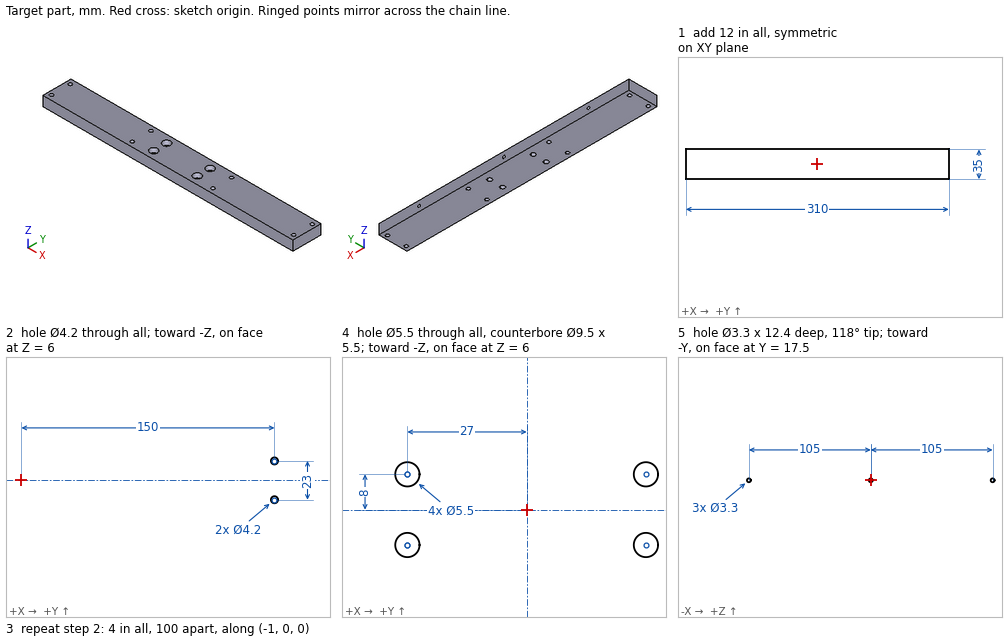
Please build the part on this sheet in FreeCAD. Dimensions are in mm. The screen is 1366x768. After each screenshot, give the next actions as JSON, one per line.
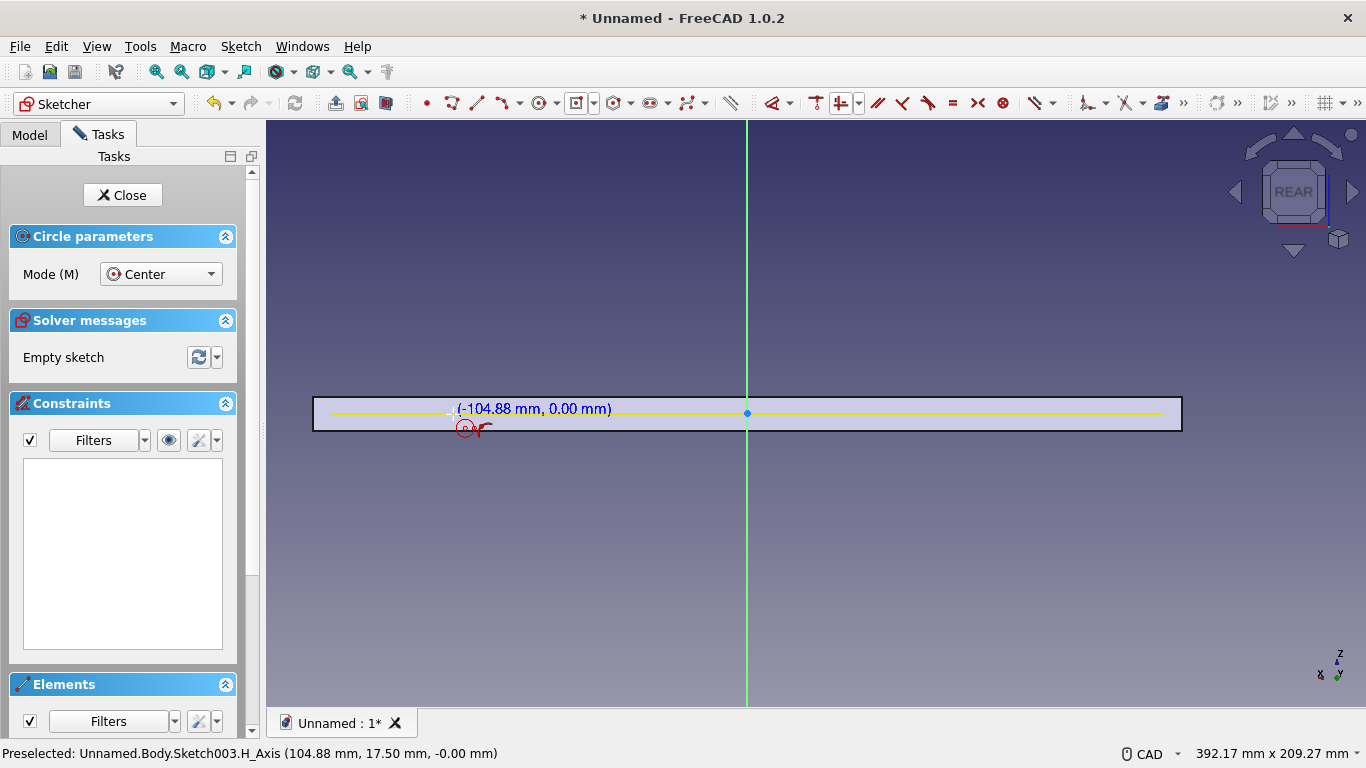
{"action": "left_click", "coordinate": [453, 414]}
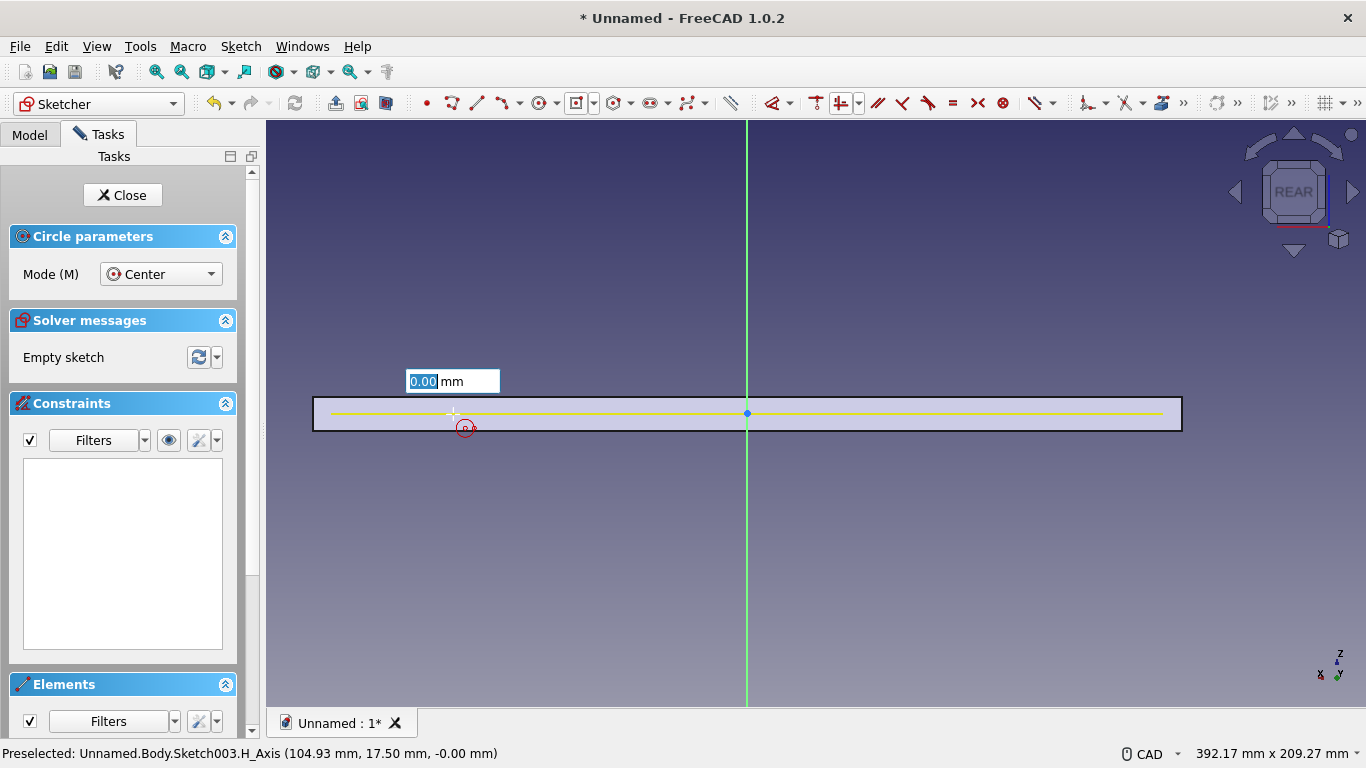
{"action": "scroll", "coordinate": [451, 418], "scroll_direction": "up", "scroll_amount": 7}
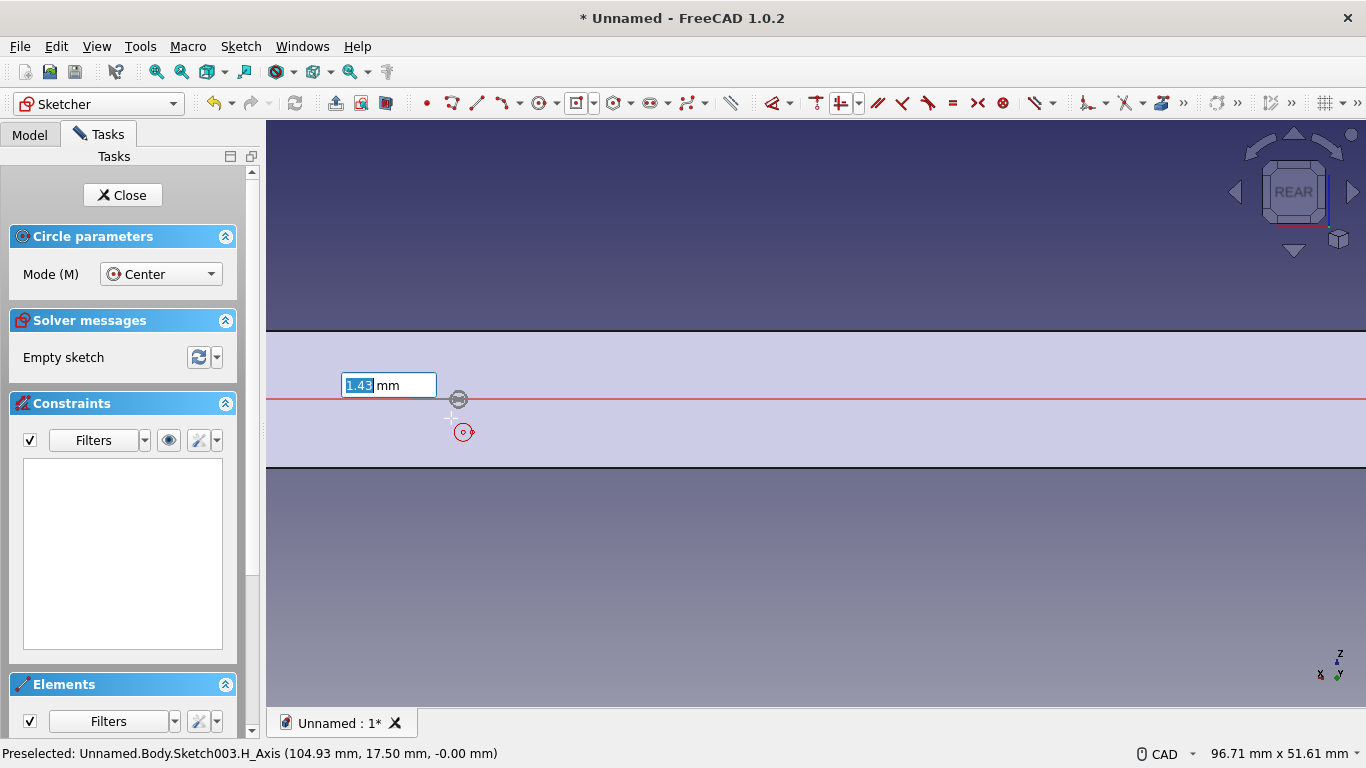
{"action": "left_click", "coordinate": [451, 417]}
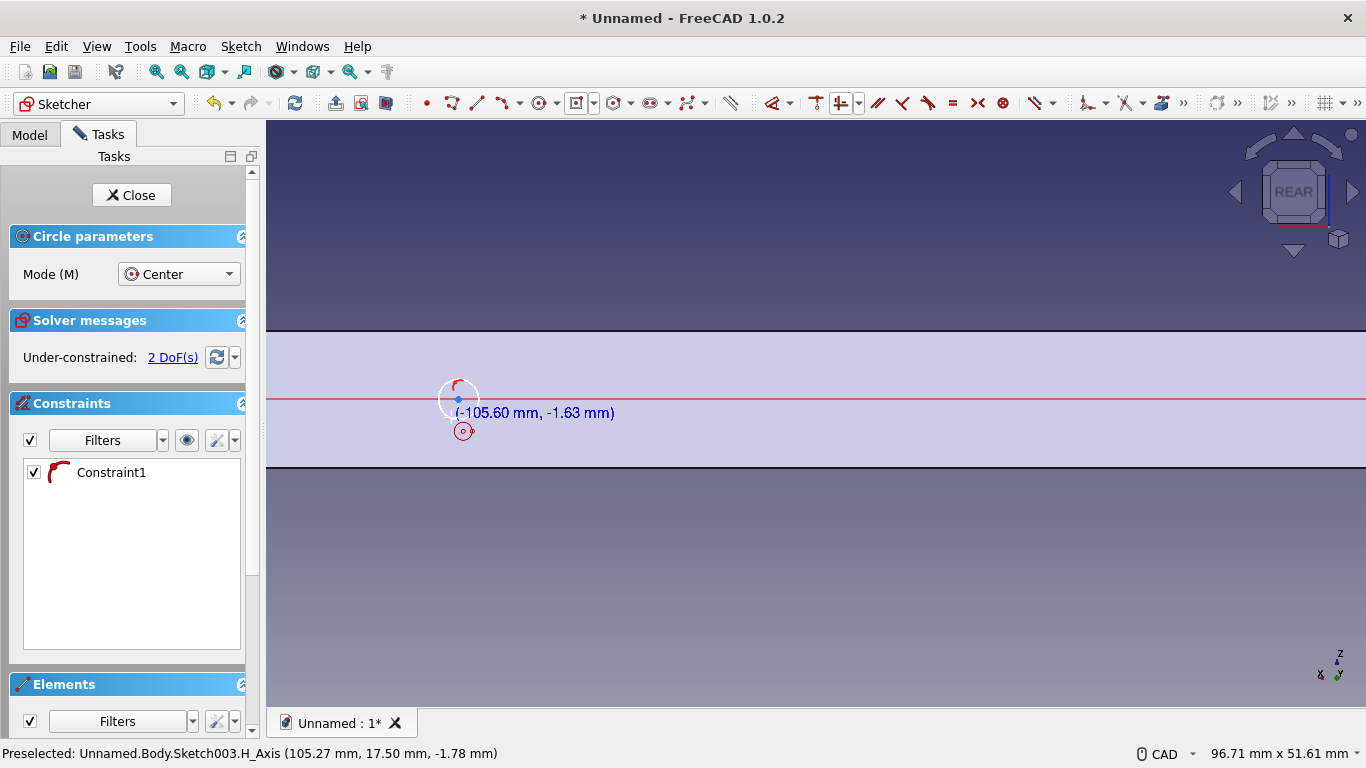
{"action": "scroll", "coordinate": [451, 418], "scroll_direction": "down", "scroll_amount": 7}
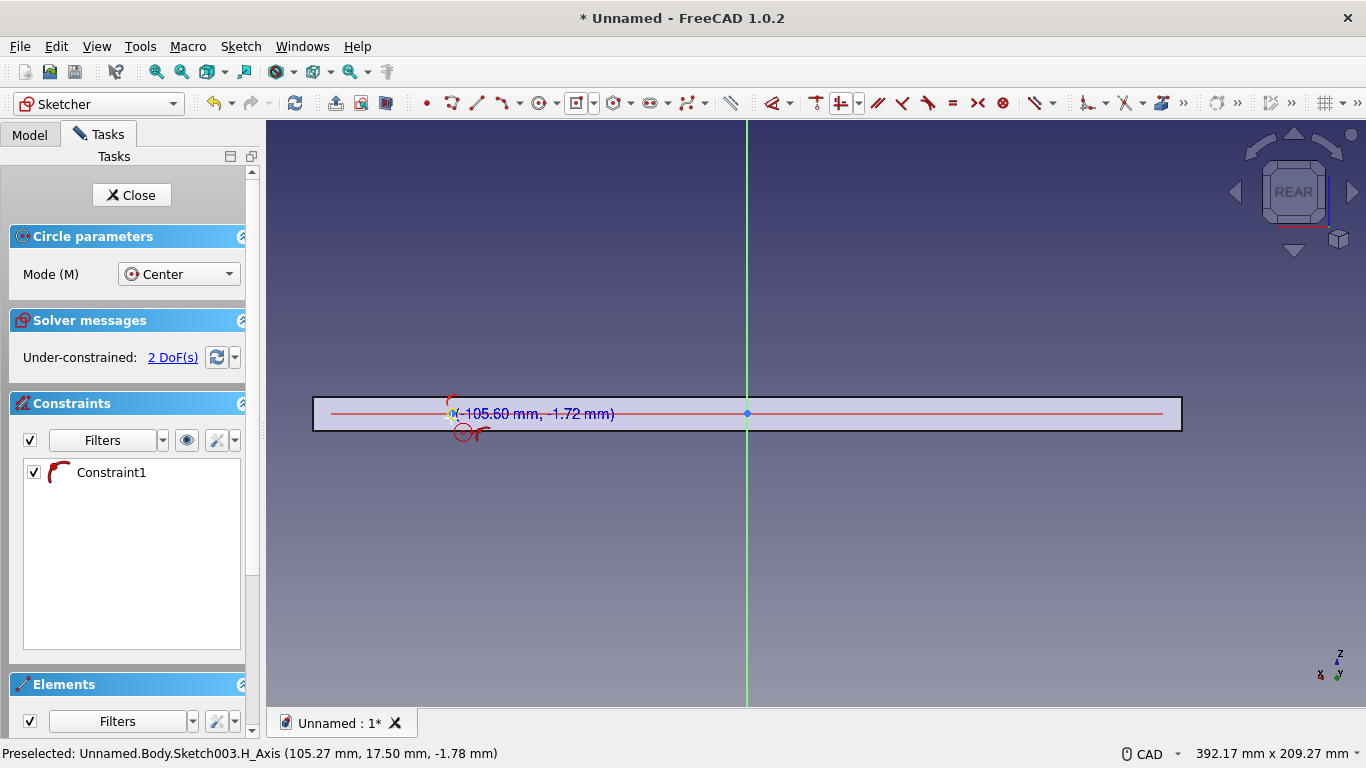
{"action": "scroll", "coordinate": [747, 414], "scroll_direction": "up", "scroll_amount": 8}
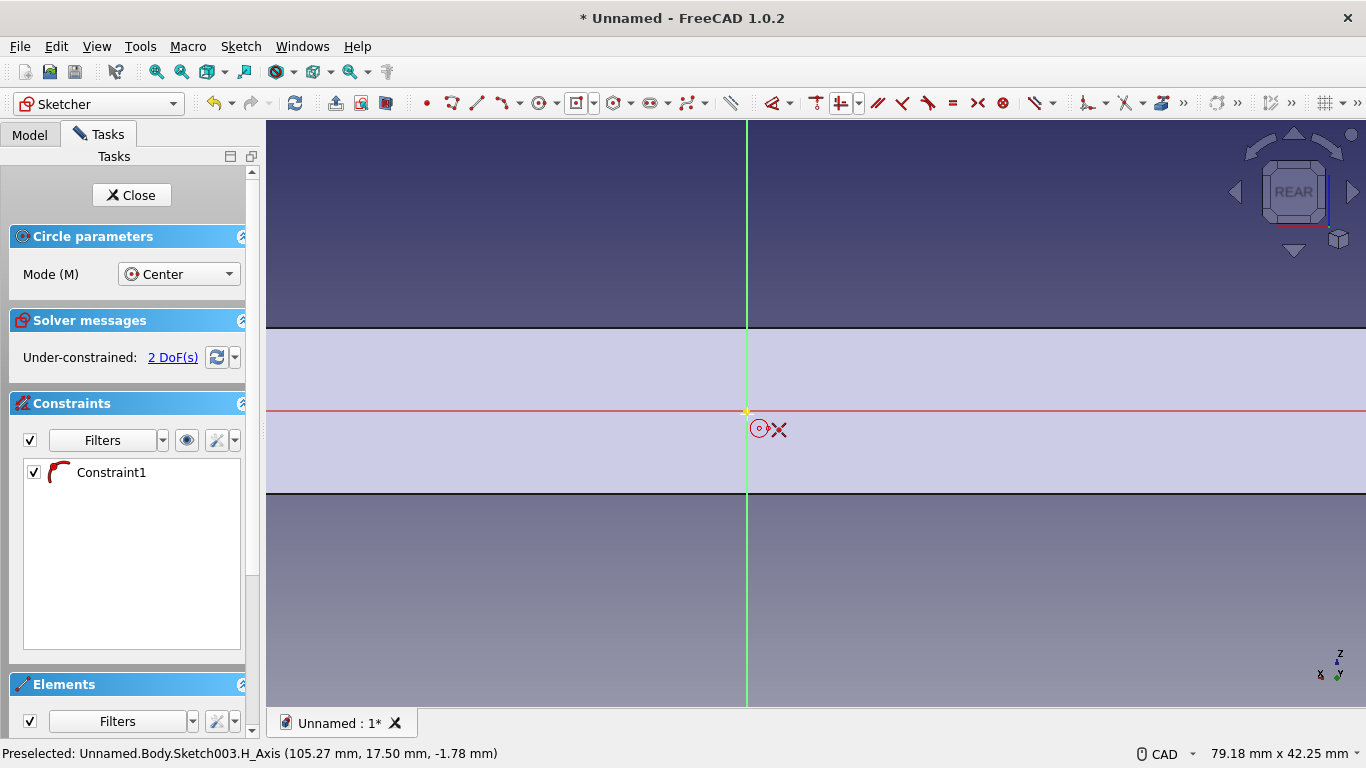
{"action": "scroll", "coordinate": [748, 414], "scroll_direction": "down", "scroll_amount": 8}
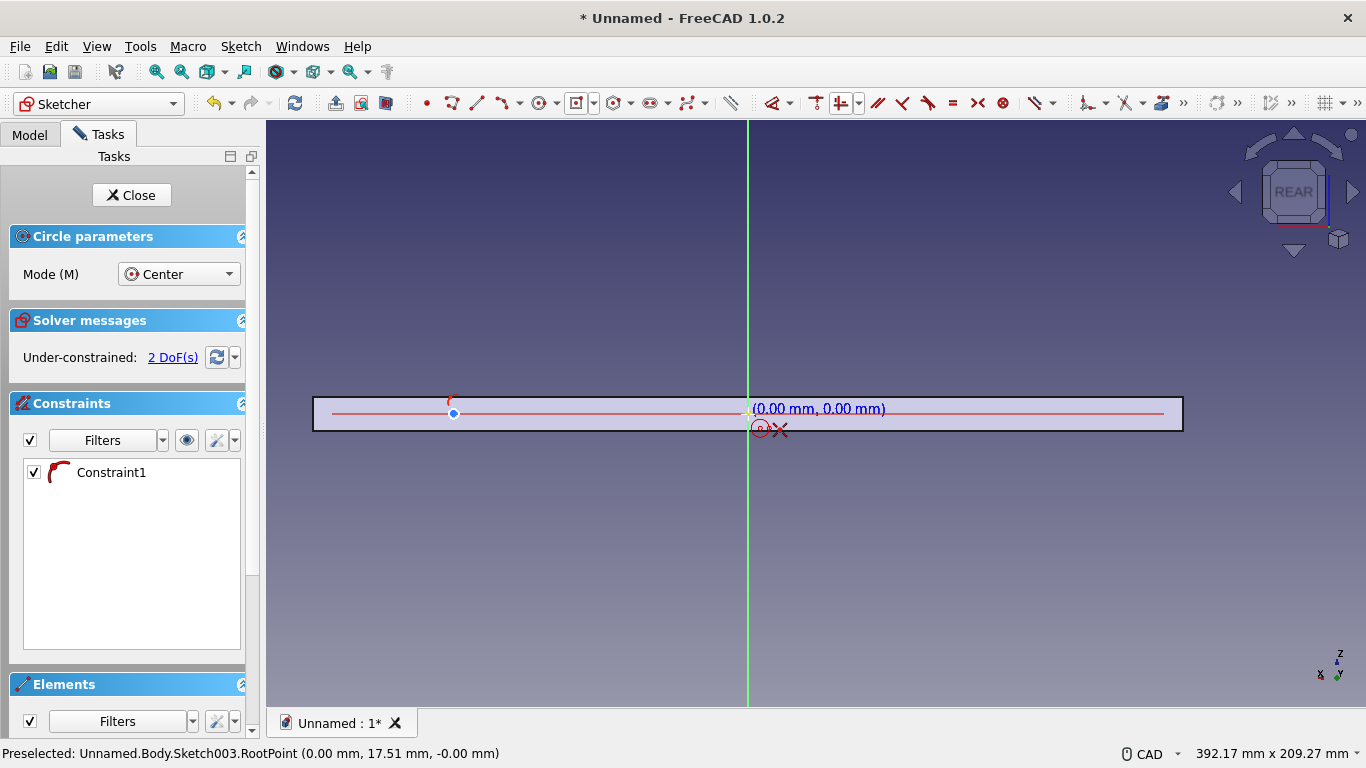
{"action": "left_click", "coordinate": [748, 414]}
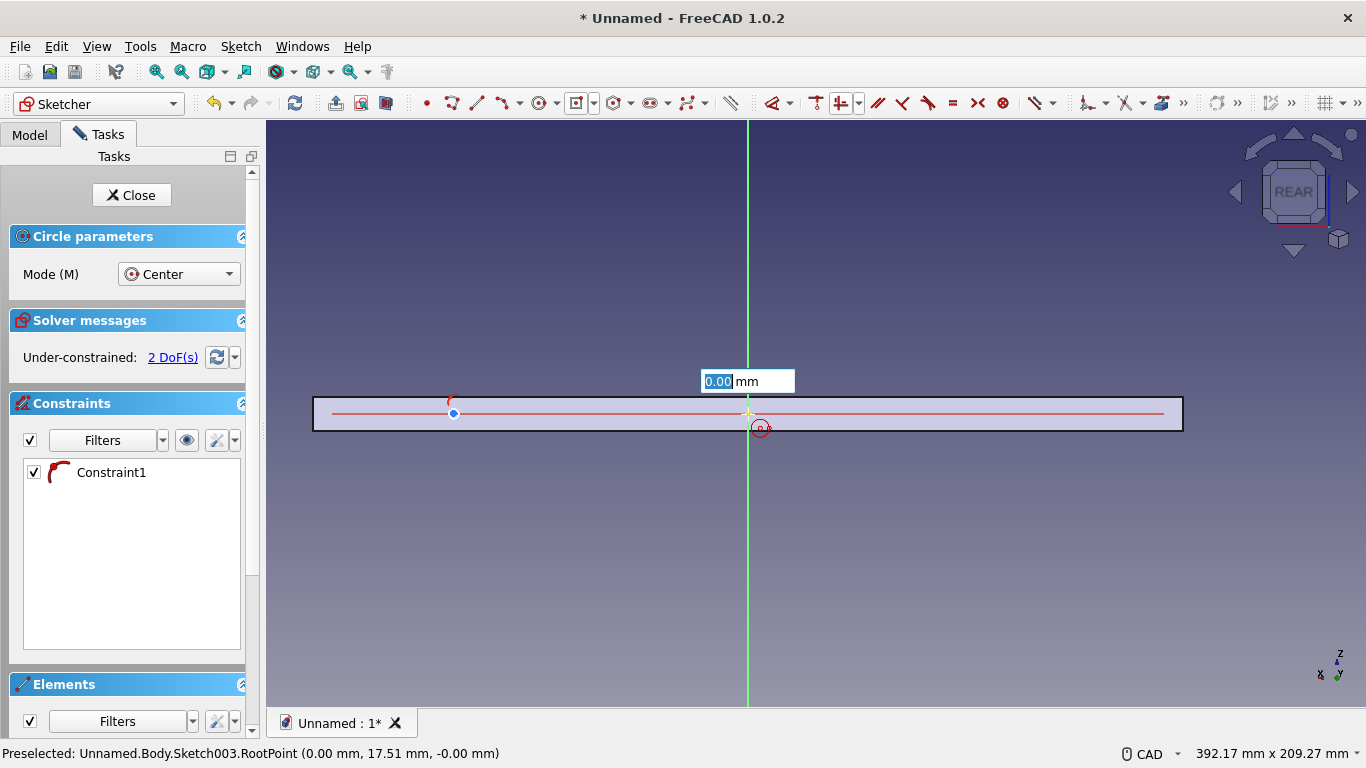
{"action": "scroll", "coordinate": [751, 411], "scroll_direction": "up", "scroll_amount": 8}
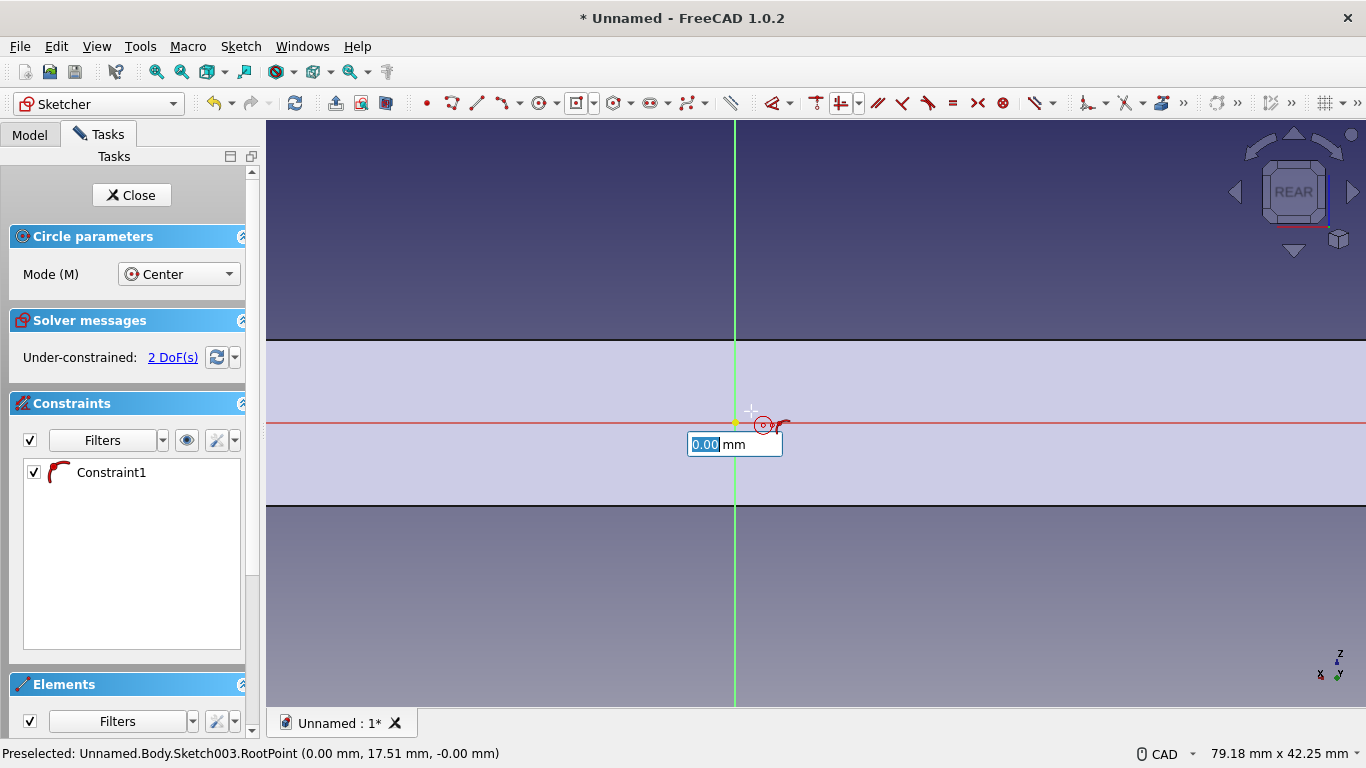
{"action": "left_click", "coordinate": [751, 407]}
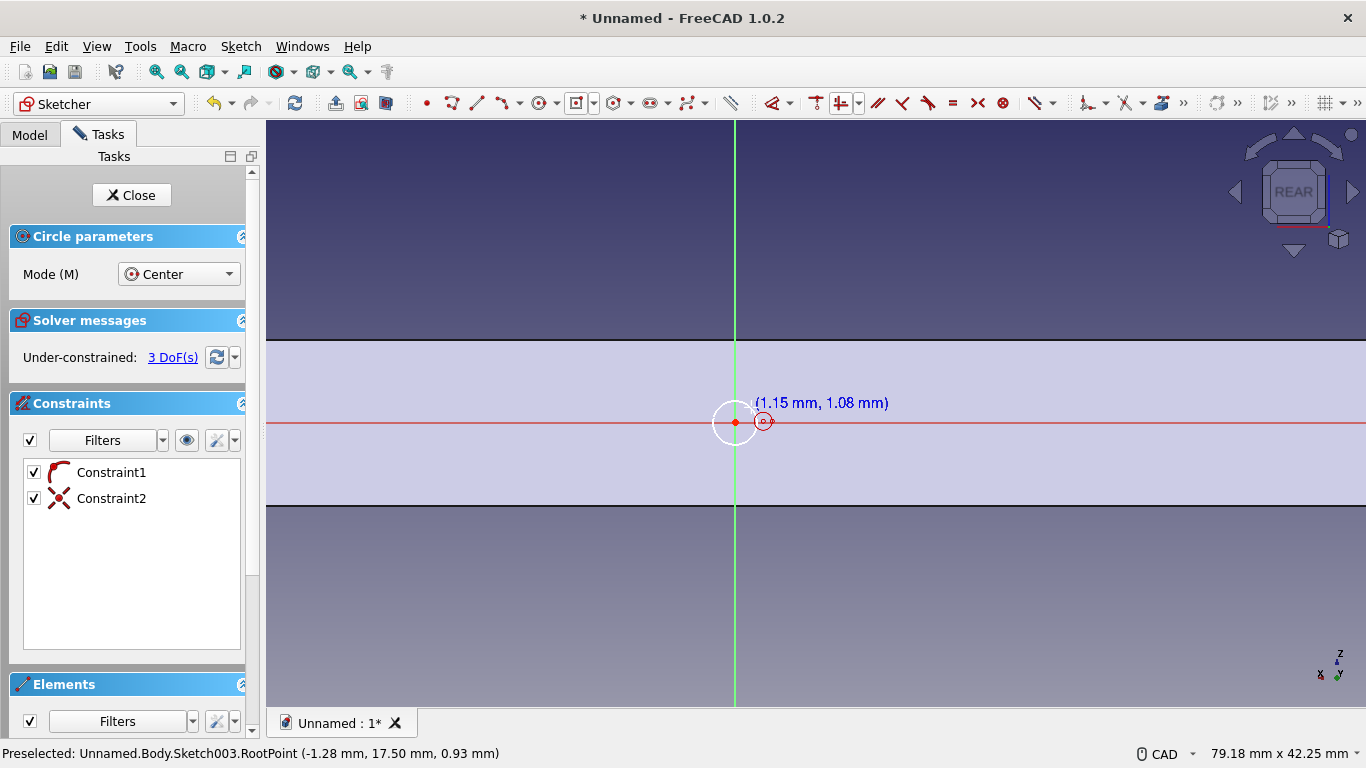
{"action": "scroll", "coordinate": [751, 411], "scroll_direction": "down", "scroll_amount": 8}